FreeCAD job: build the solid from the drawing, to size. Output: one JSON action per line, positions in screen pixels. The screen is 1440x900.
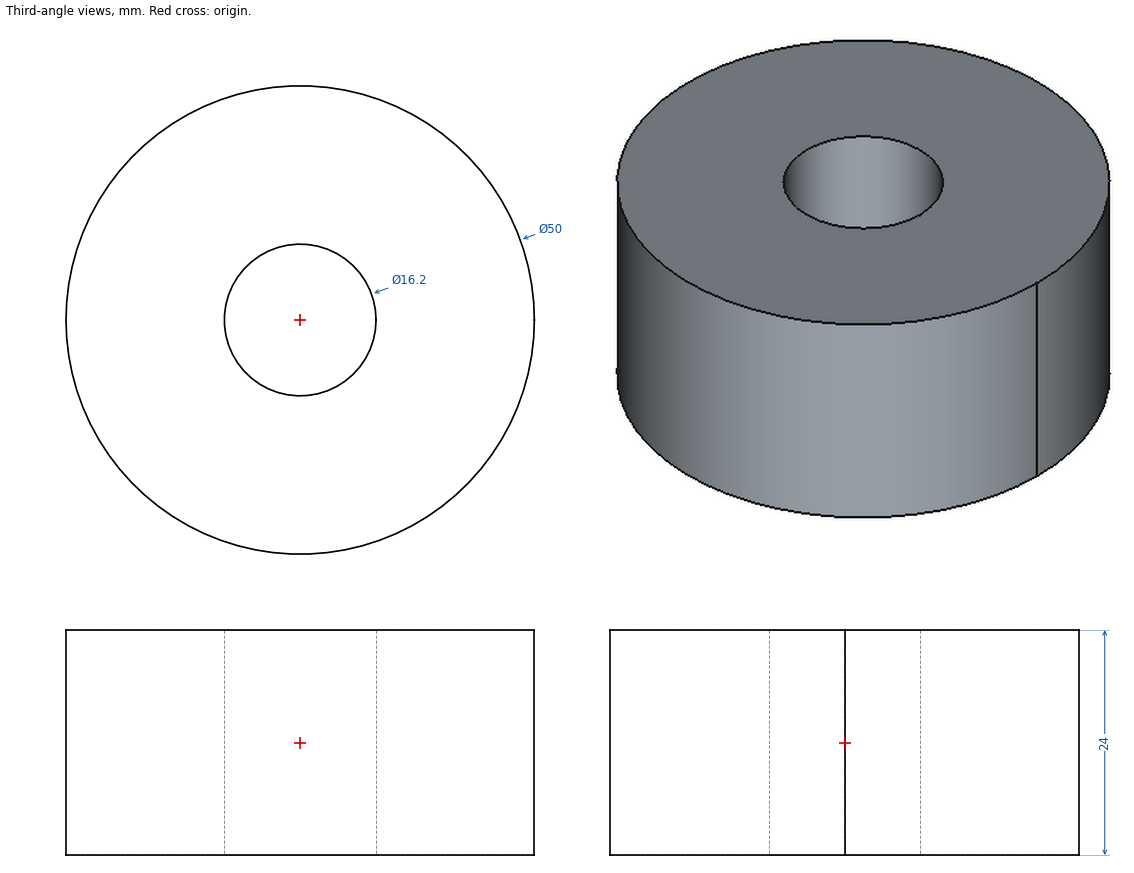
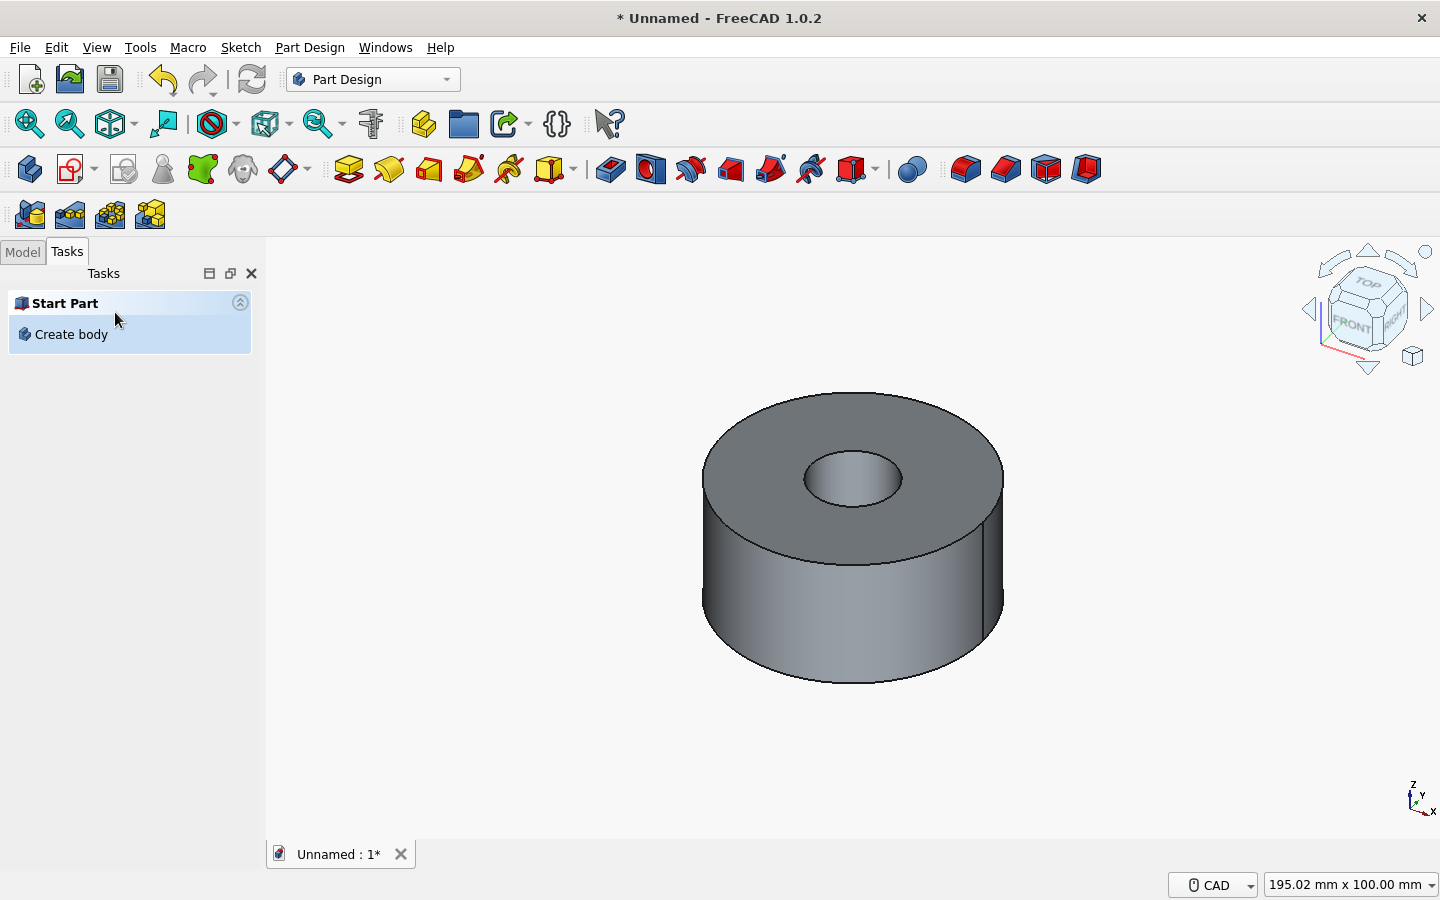
{"action": "key", "text": "0"}